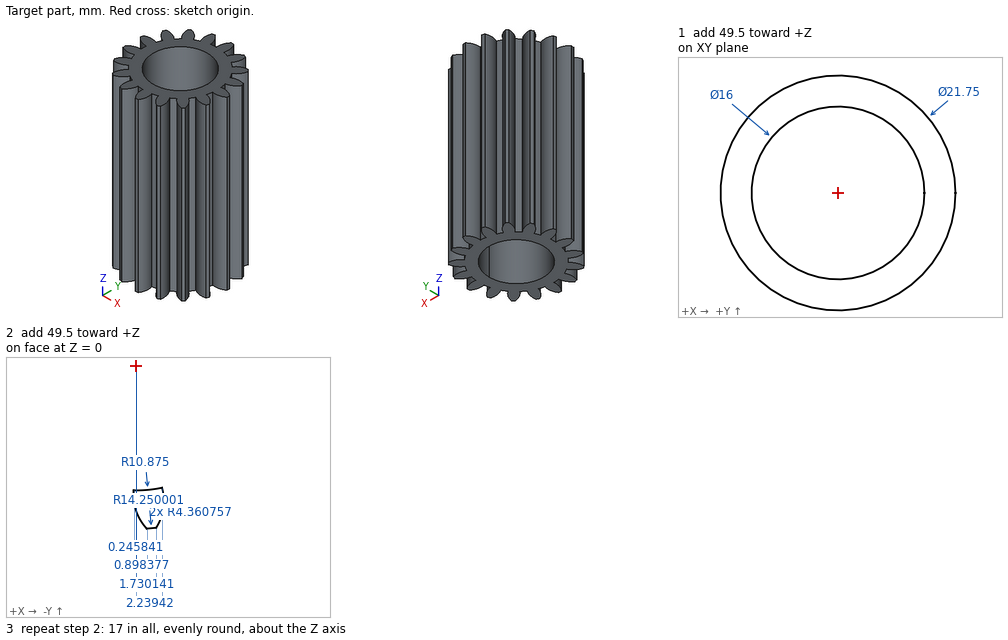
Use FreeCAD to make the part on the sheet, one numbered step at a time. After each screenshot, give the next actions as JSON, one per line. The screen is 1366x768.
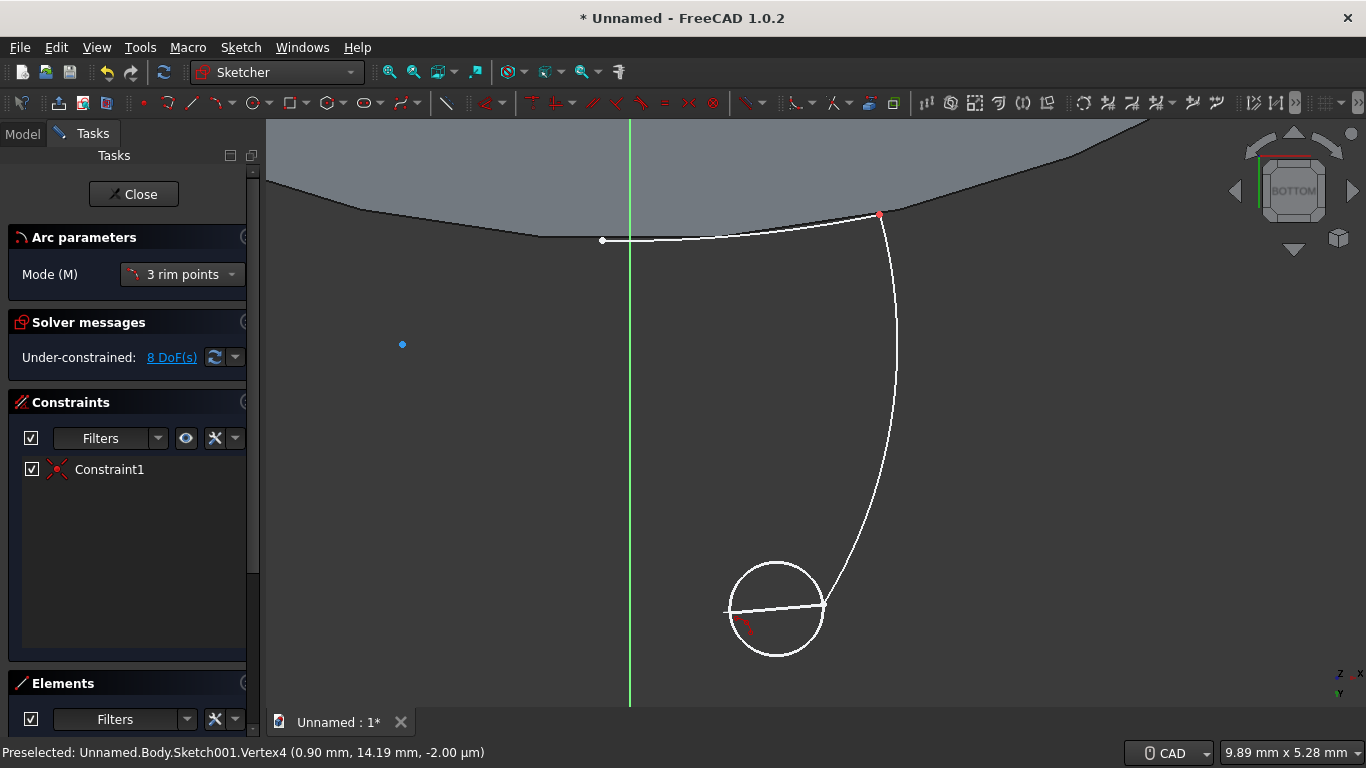
{"action": "scroll", "coordinate": [777, 609], "scroll_direction": "up", "scroll_amount": 16}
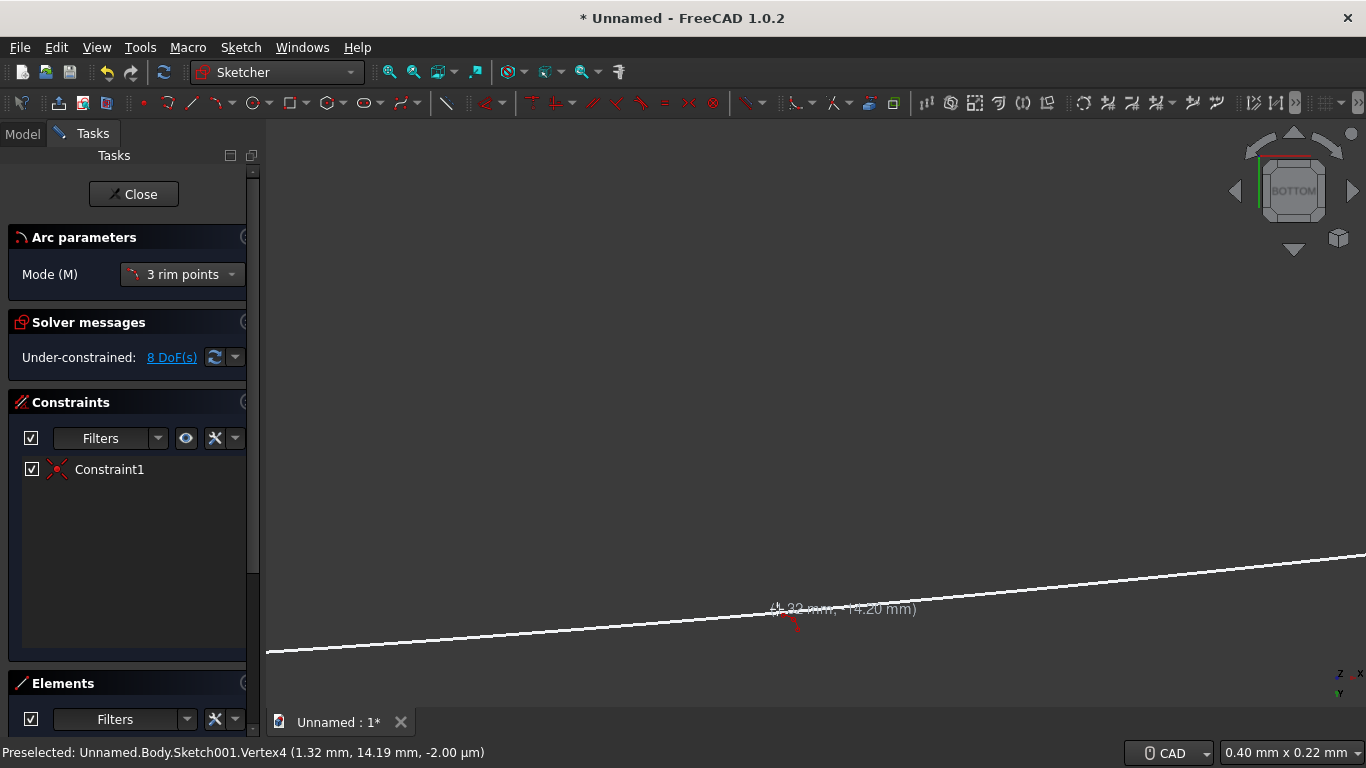
{"action": "left_click", "coordinate": [756, 586]}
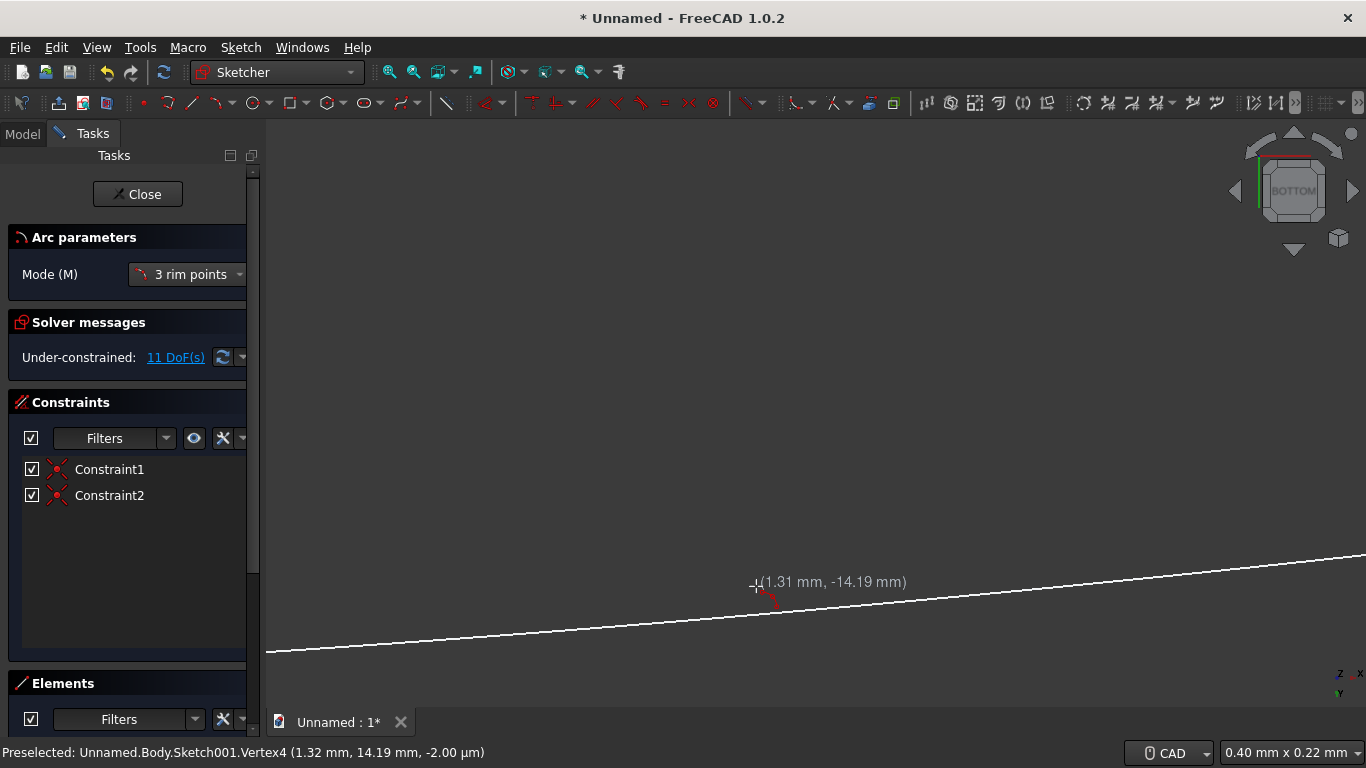
{"action": "scroll", "coordinate": [777, 609], "scroll_direction": "down", "scroll_amount": 16}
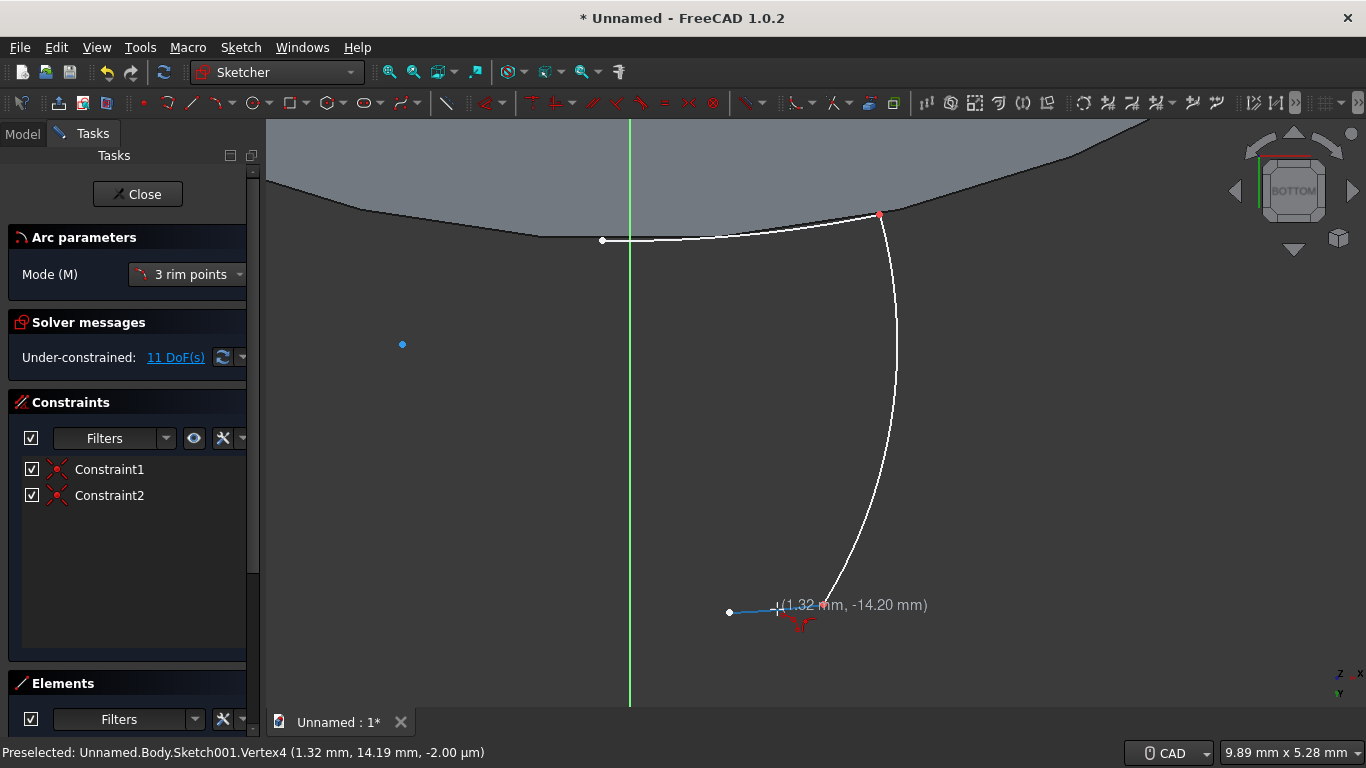
{"action": "left_click", "coordinate": [730, 613]}
{"action": "left_click", "coordinate": [603, 241]}
{"action": "left_click", "coordinate": [616, 401]}
{"action": "key", "text": "Escape"}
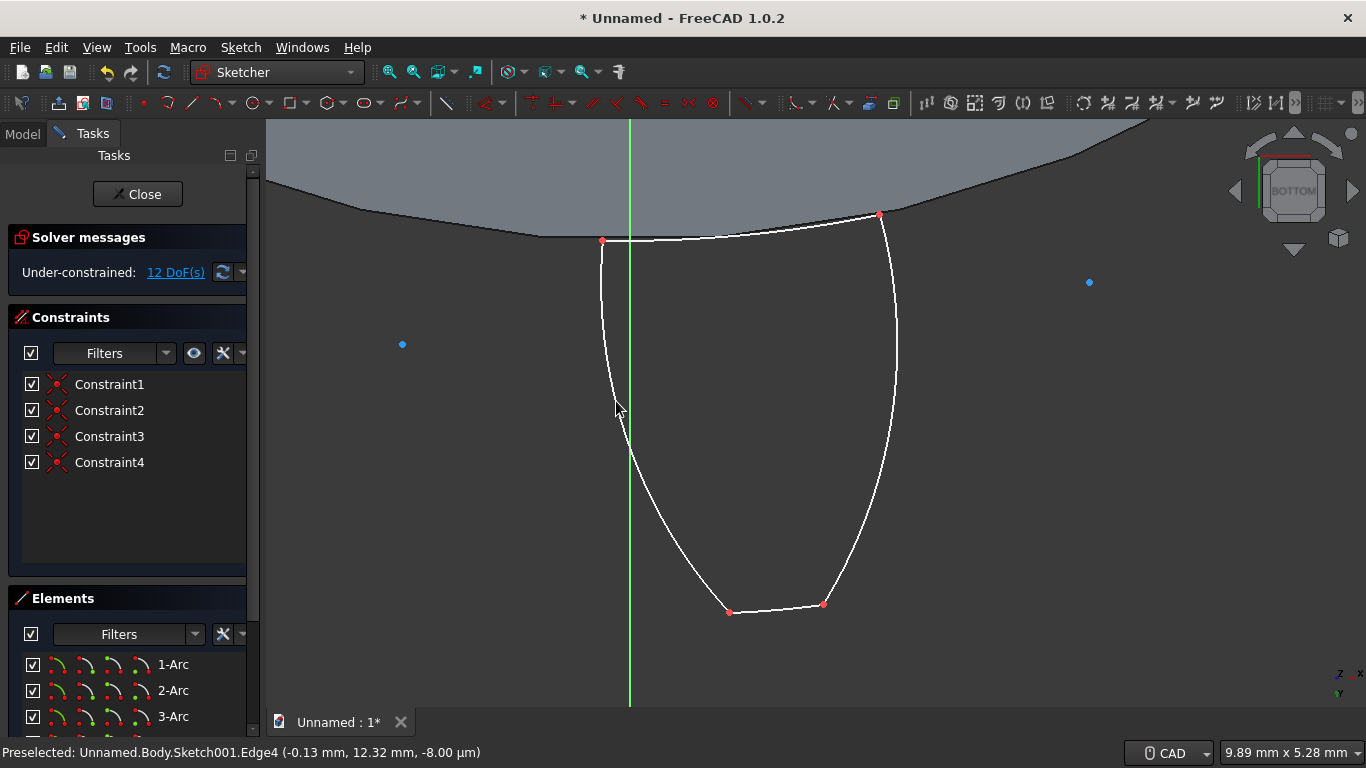
{"action": "left_click", "coordinate": [687, 239]}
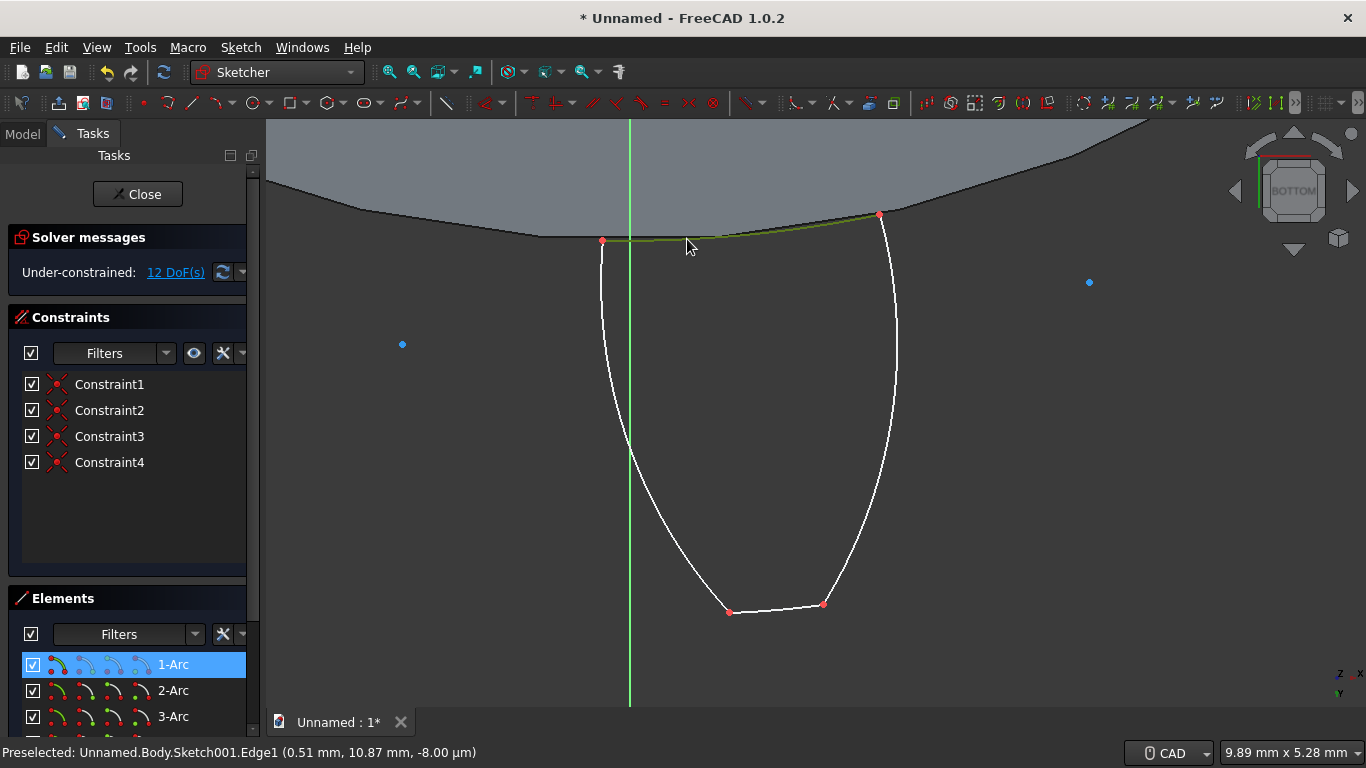
{"action": "left_click", "coordinate": [758, 611]}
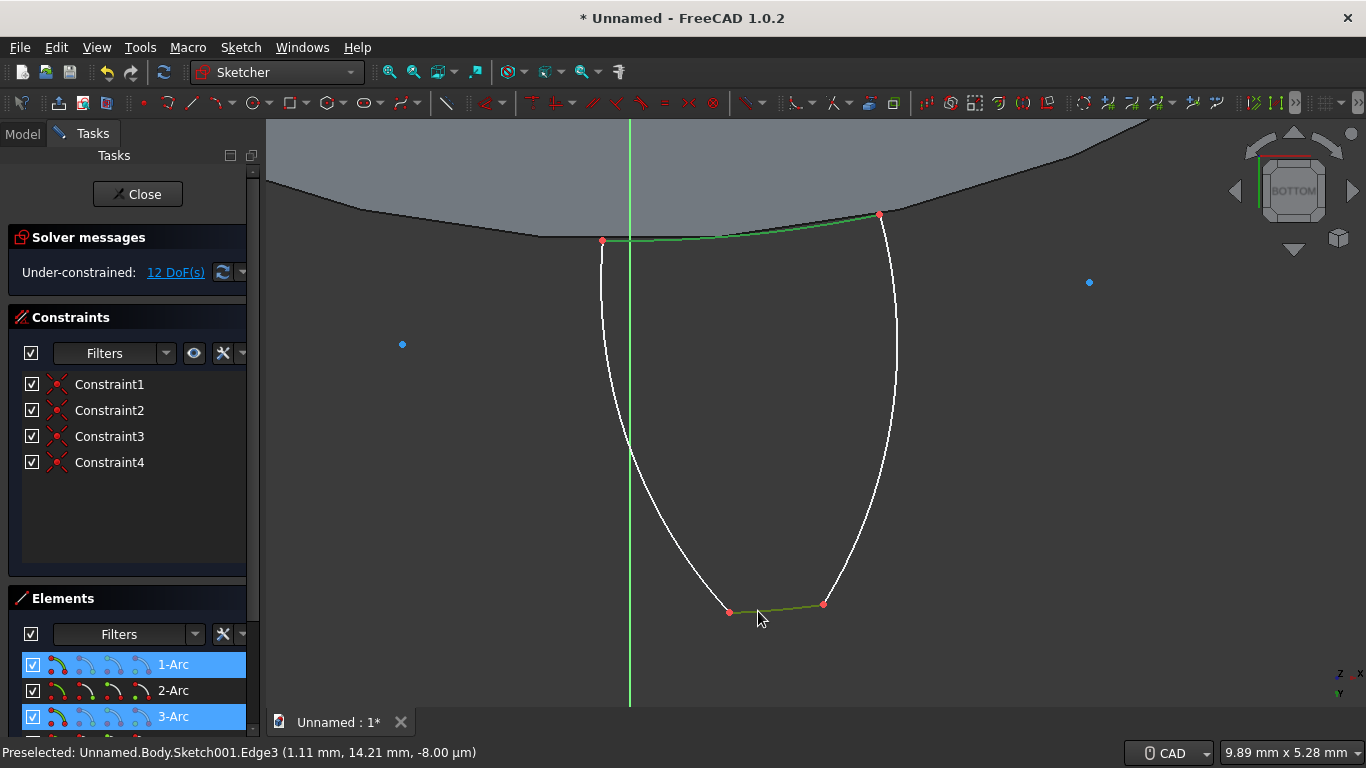
{"action": "left_click", "coordinate": [532, 104]}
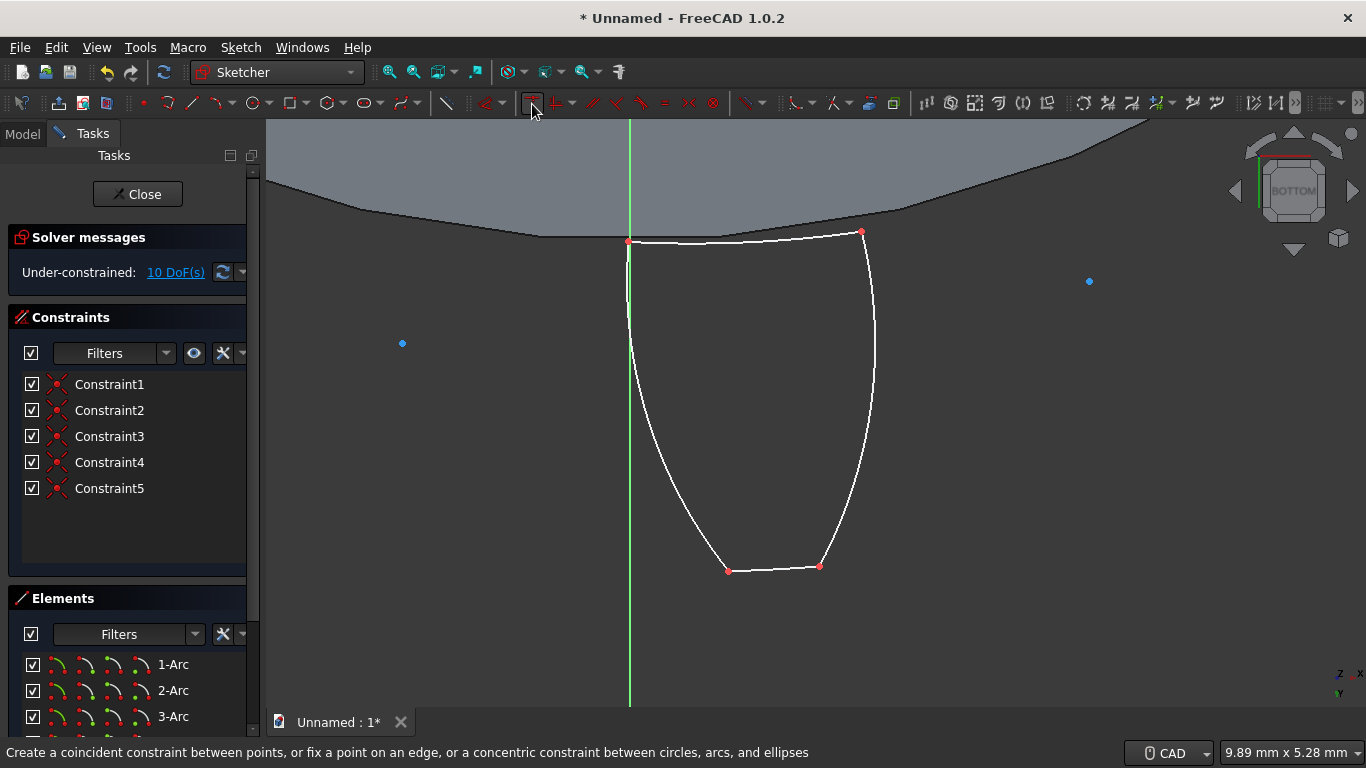
{"action": "scroll", "coordinate": [747, 606], "scroll_direction": "down", "scroll_amount": 7}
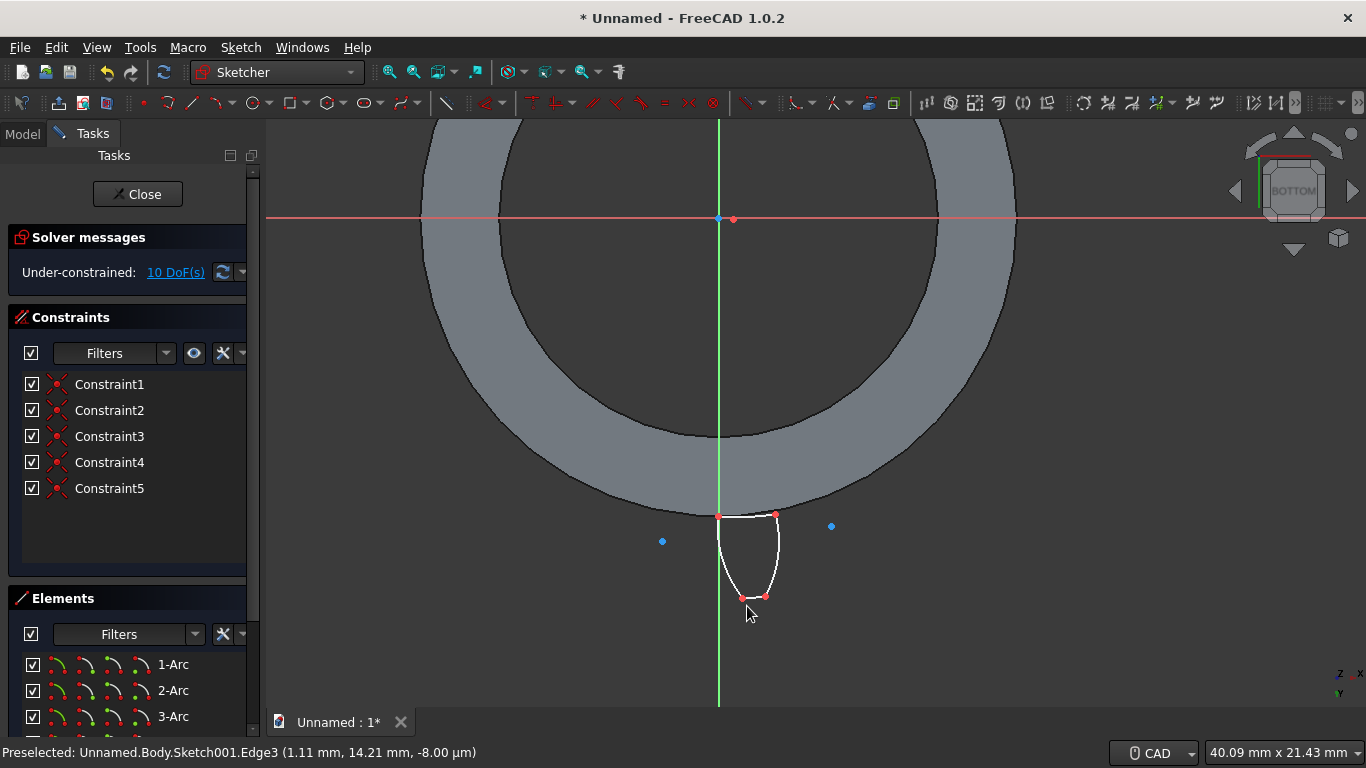
{"action": "left_click_drag", "start_coordinate": [709, 208], "coordinate": [744, 230]}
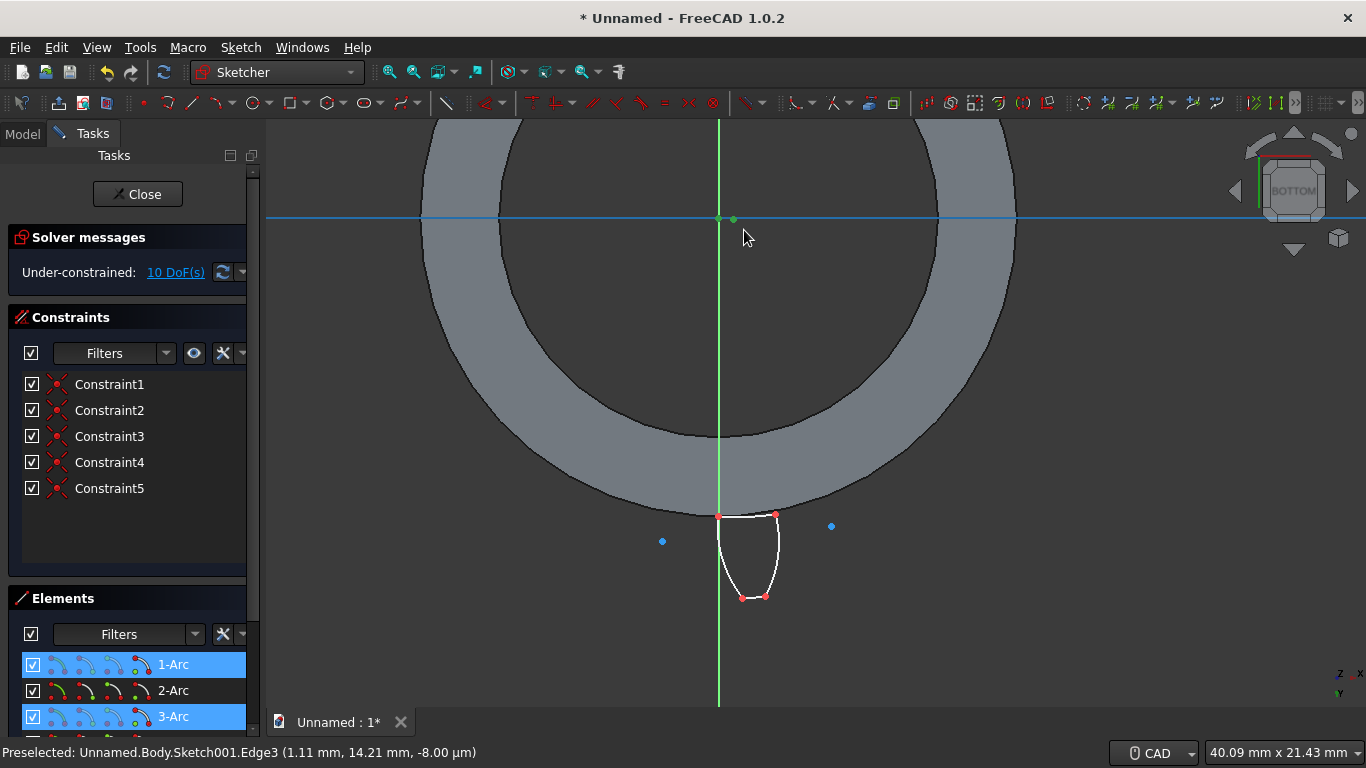
{"action": "left_click", "coordinate": [532, 104]}